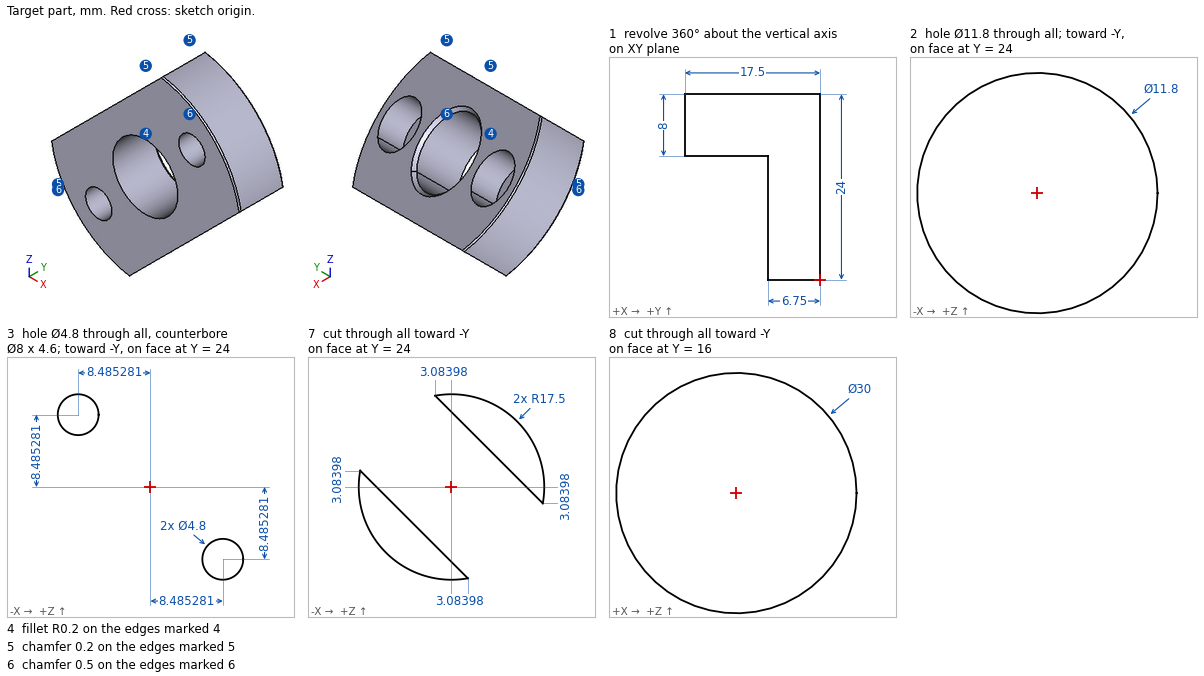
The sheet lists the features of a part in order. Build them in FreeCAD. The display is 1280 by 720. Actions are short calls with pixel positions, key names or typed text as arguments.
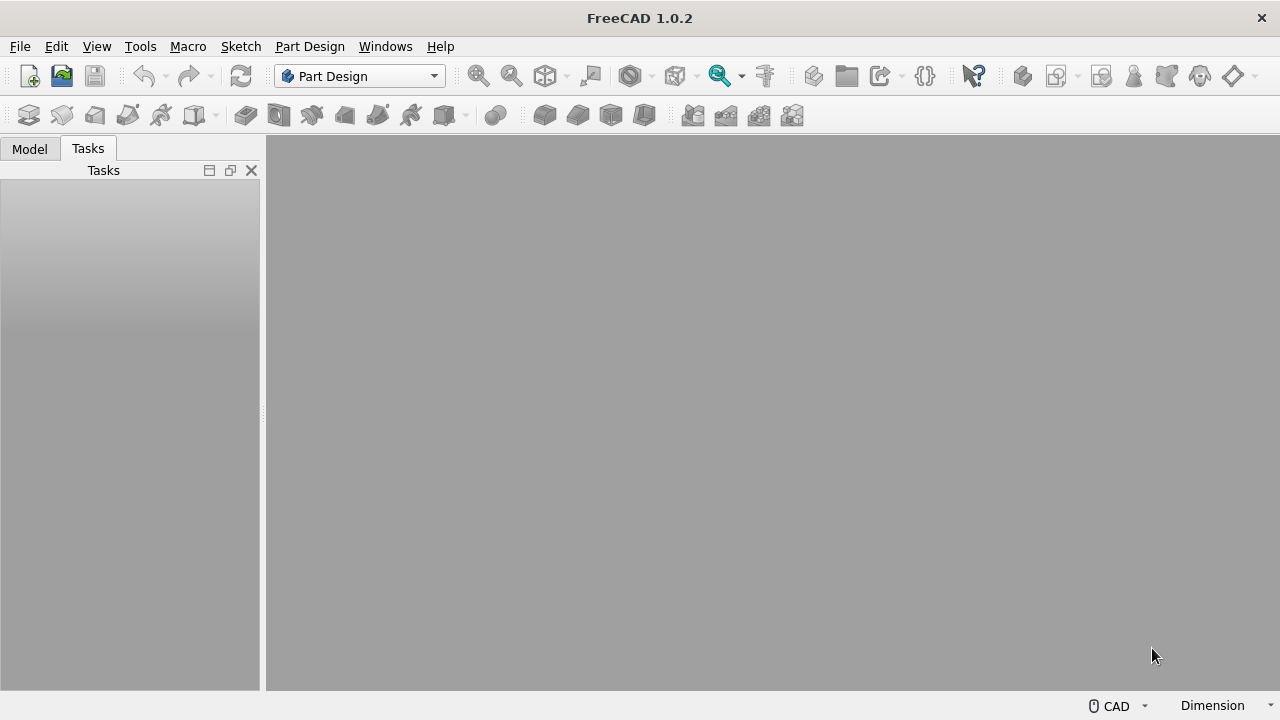
click(29, 76)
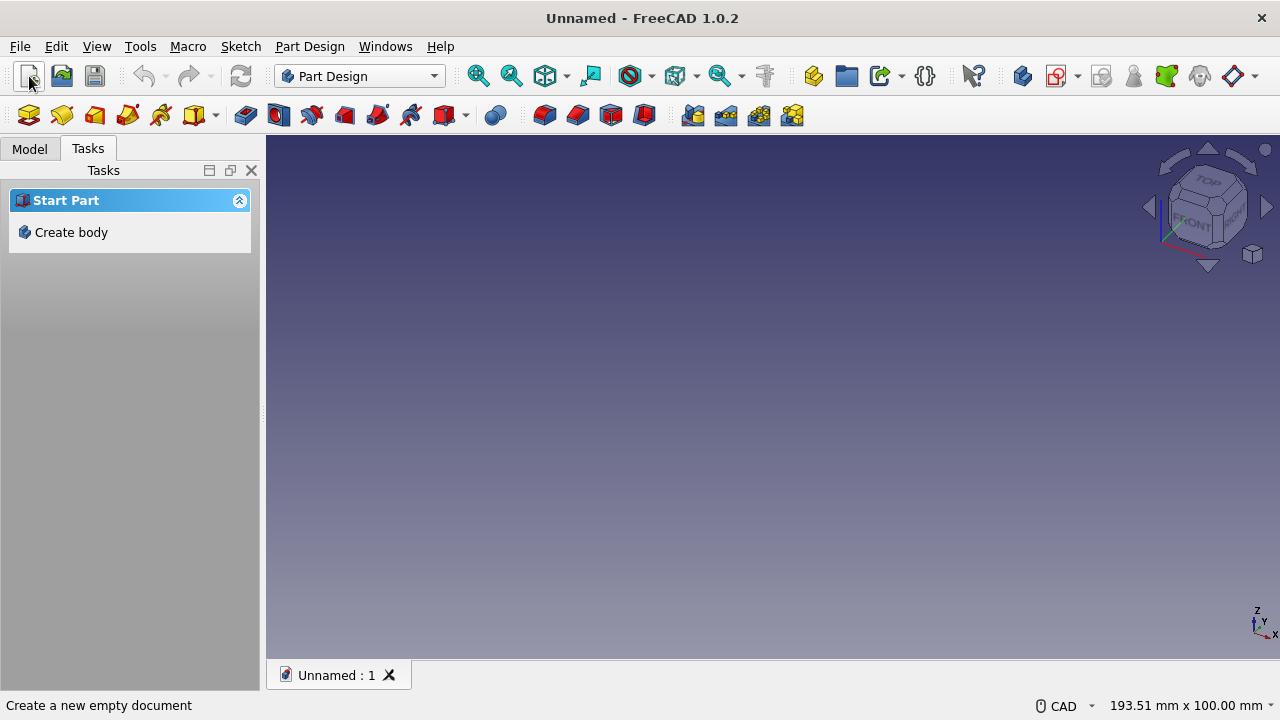
click(1056, 76)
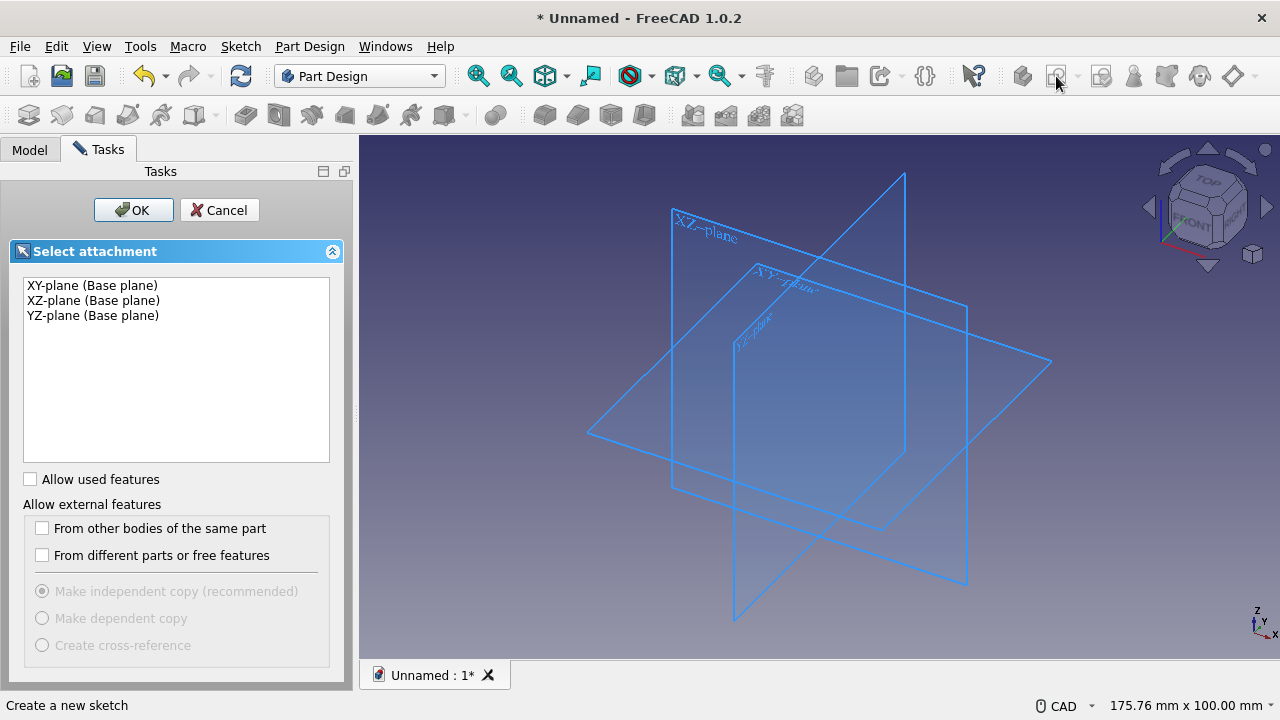
click(84, 286)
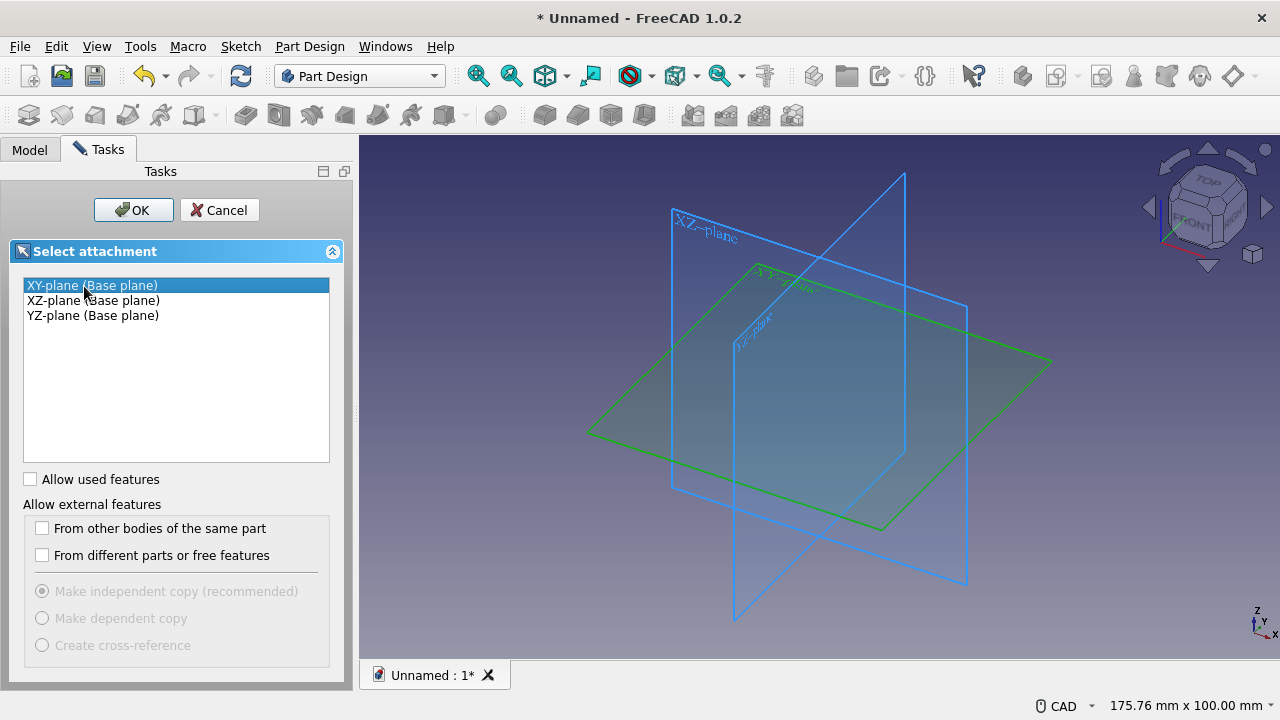
click(134, 210)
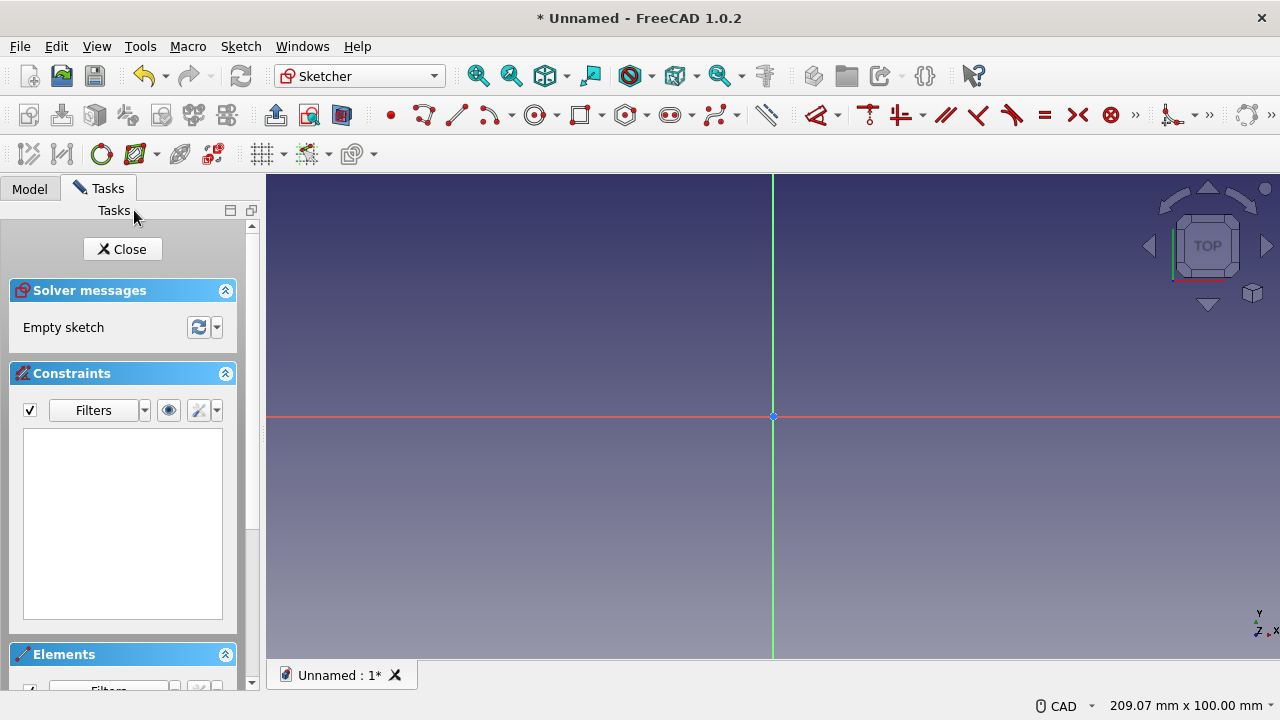
scroll(746, 324, up, 5)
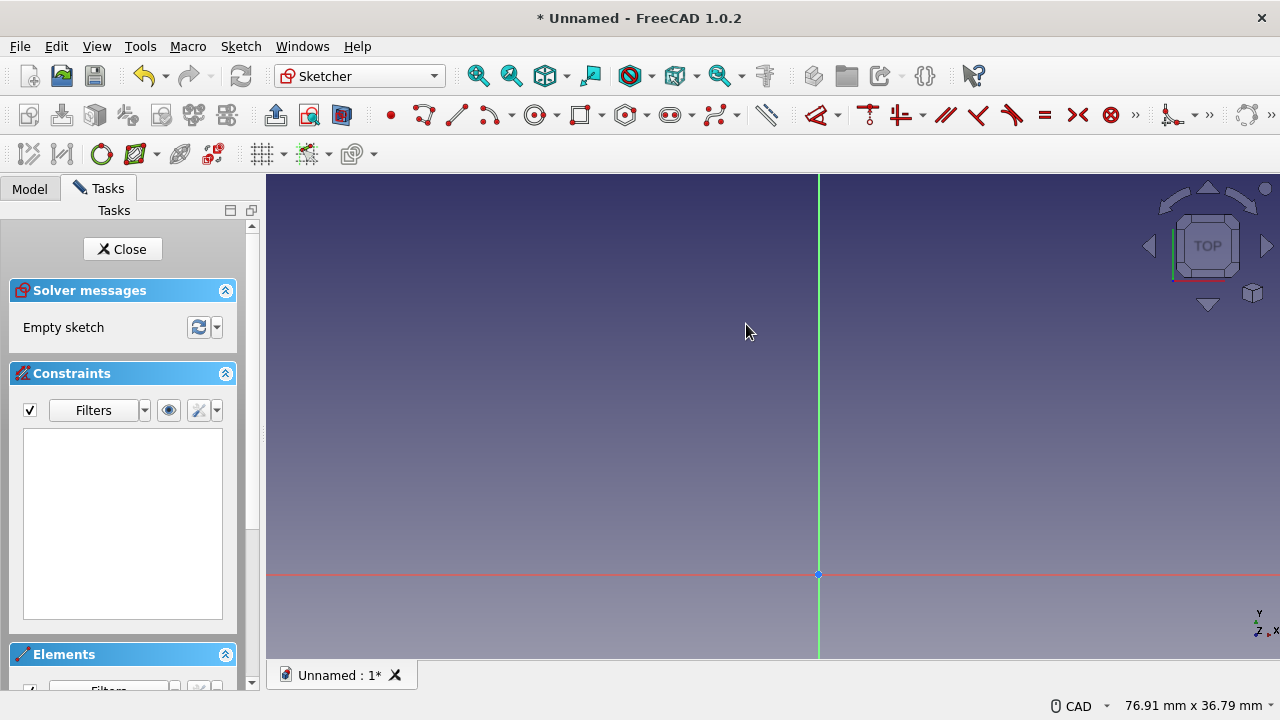
key(g)
key(m)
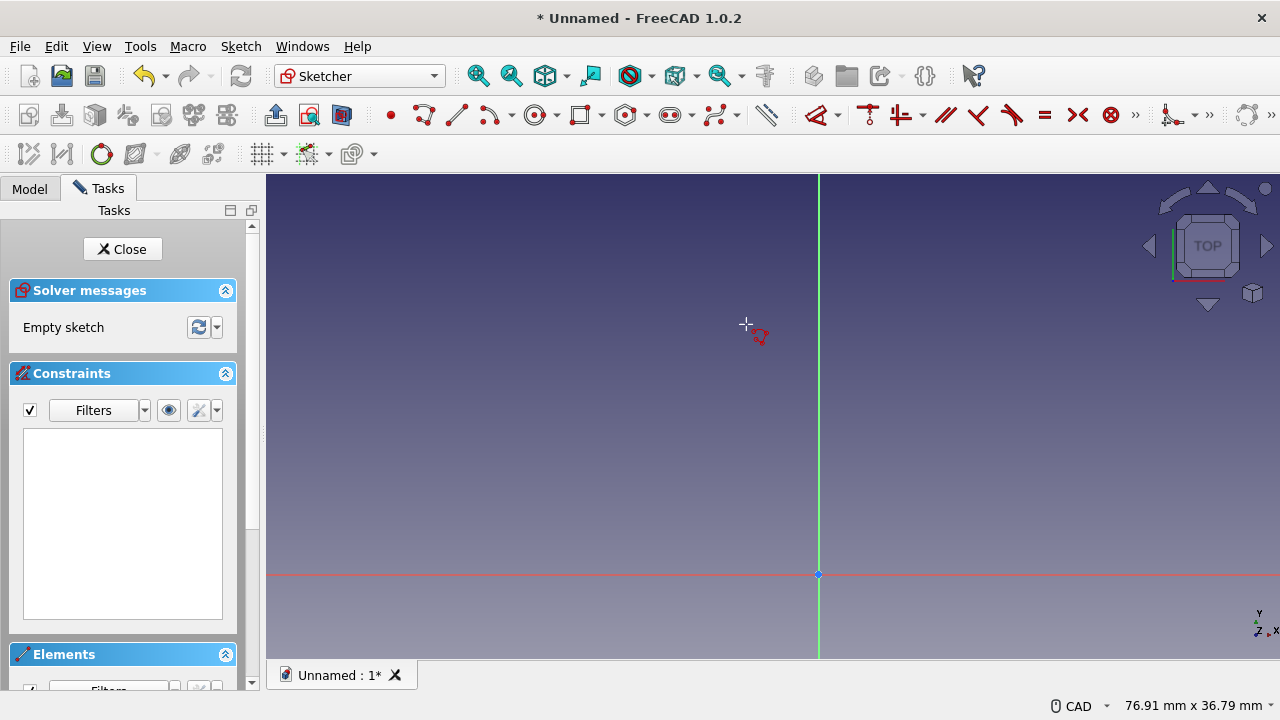
click(819, 575)
click(810, 259)
click(588, 259)
click(588, 364)
click(730, 364)
click(730, 566)
click(819, 575)
key(Escape)
key(Escape)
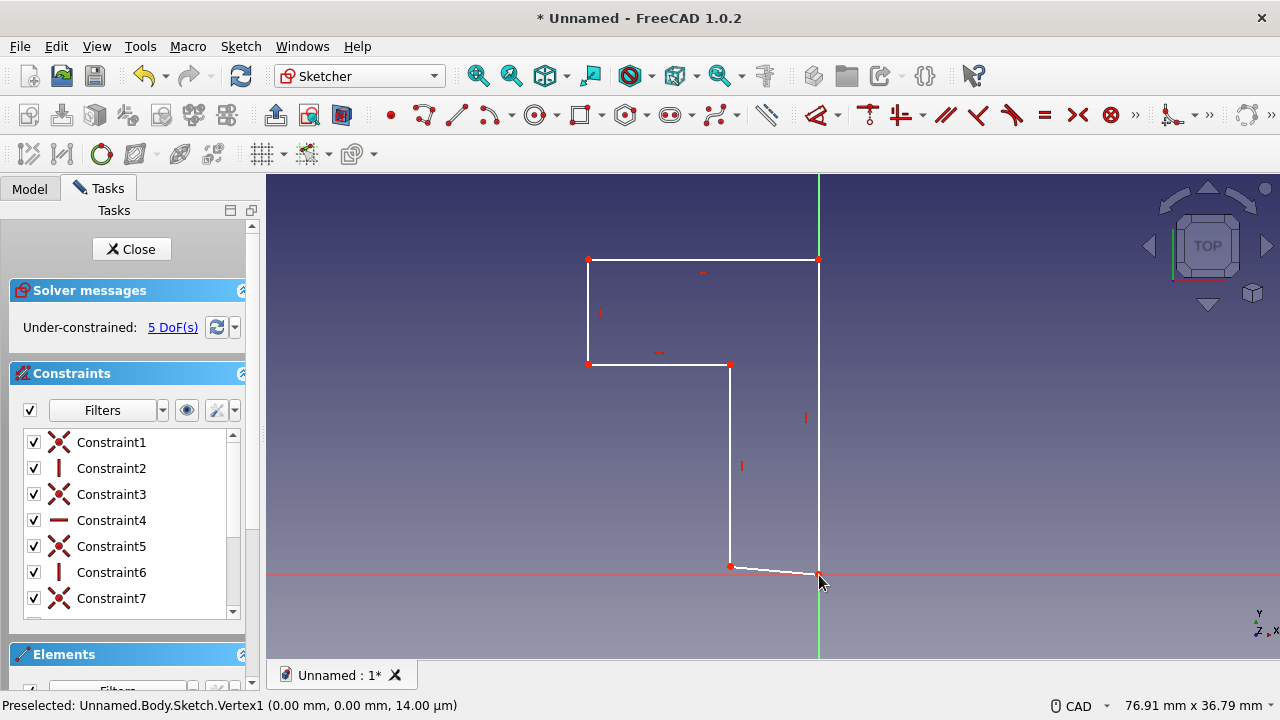
click(792, 573)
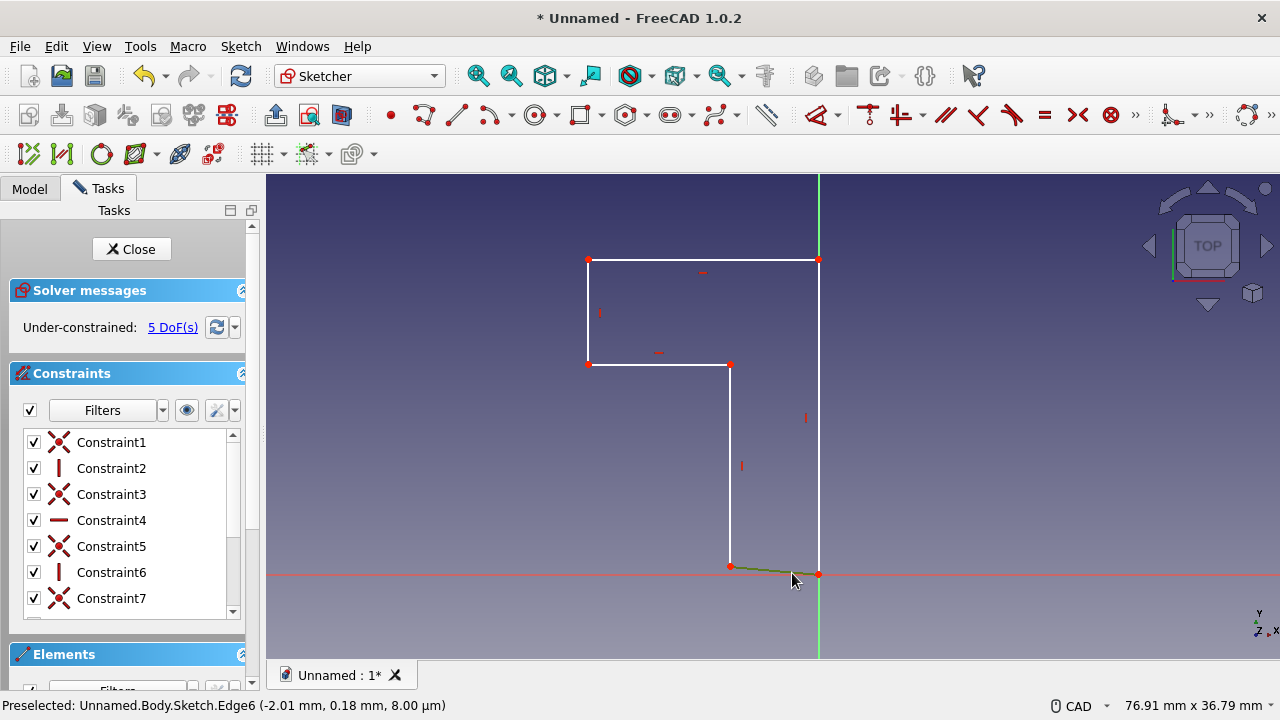
key(h)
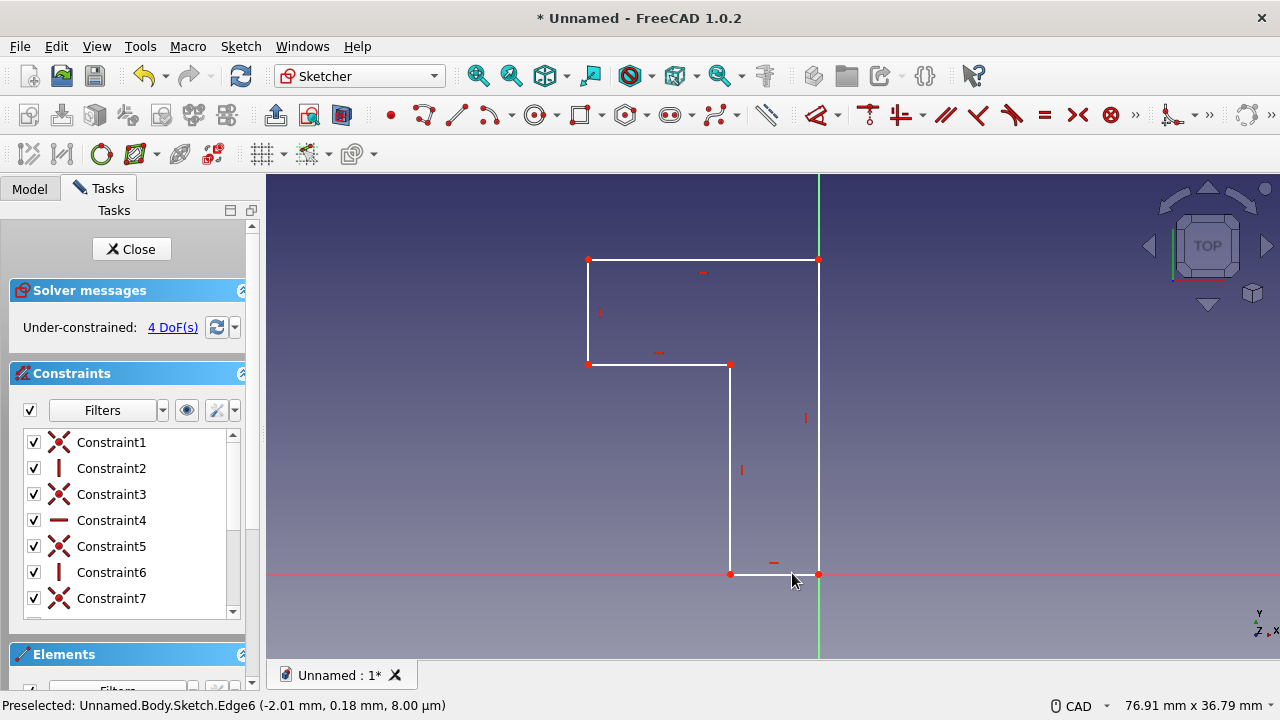
click(588, 291)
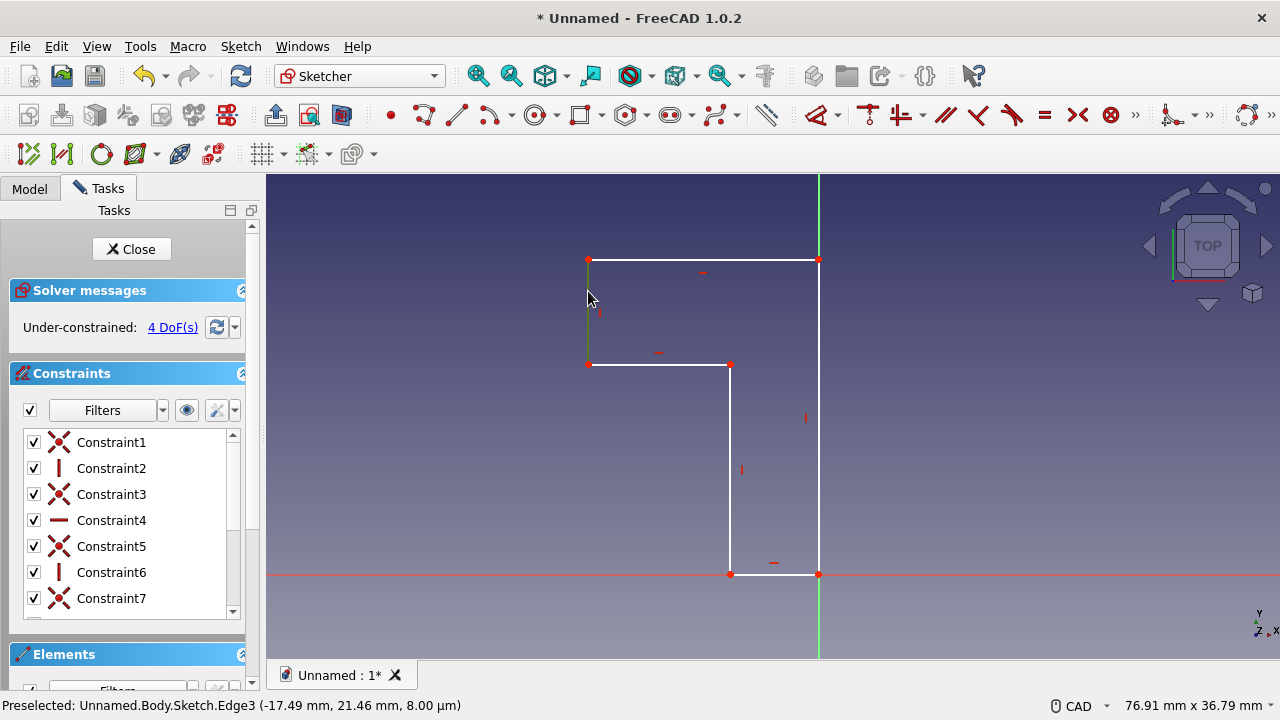
key(i)